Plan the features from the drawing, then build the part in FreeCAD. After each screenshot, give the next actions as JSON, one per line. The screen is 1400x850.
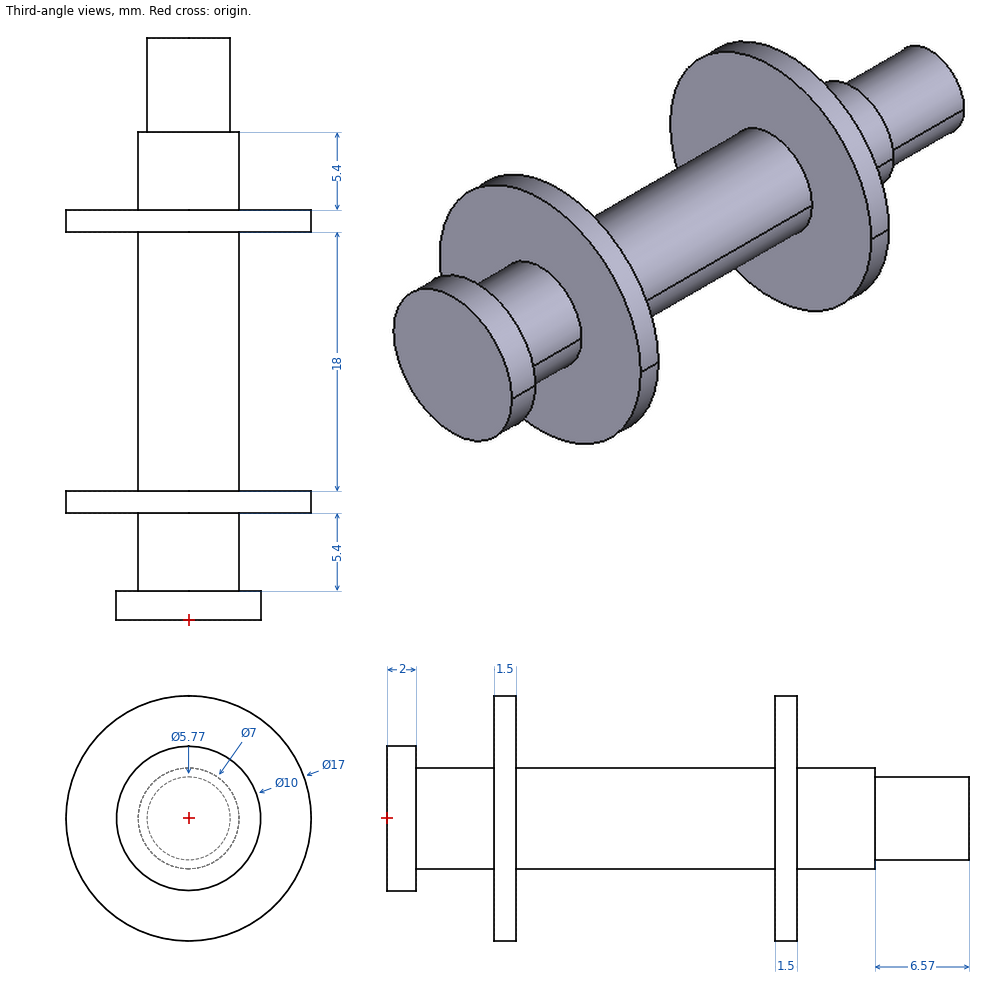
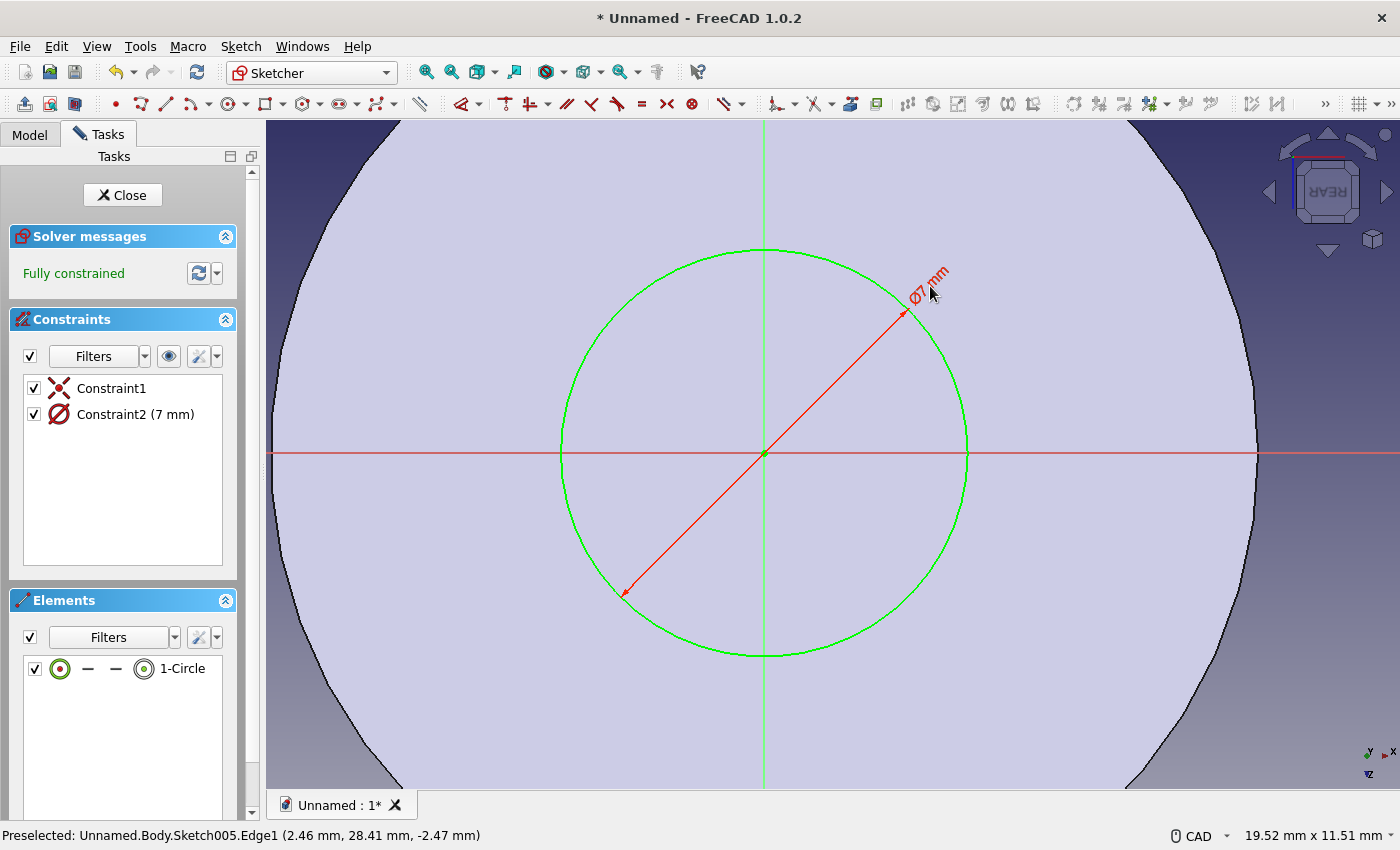
{"action": "left_click", "coordinate": [123, 195]}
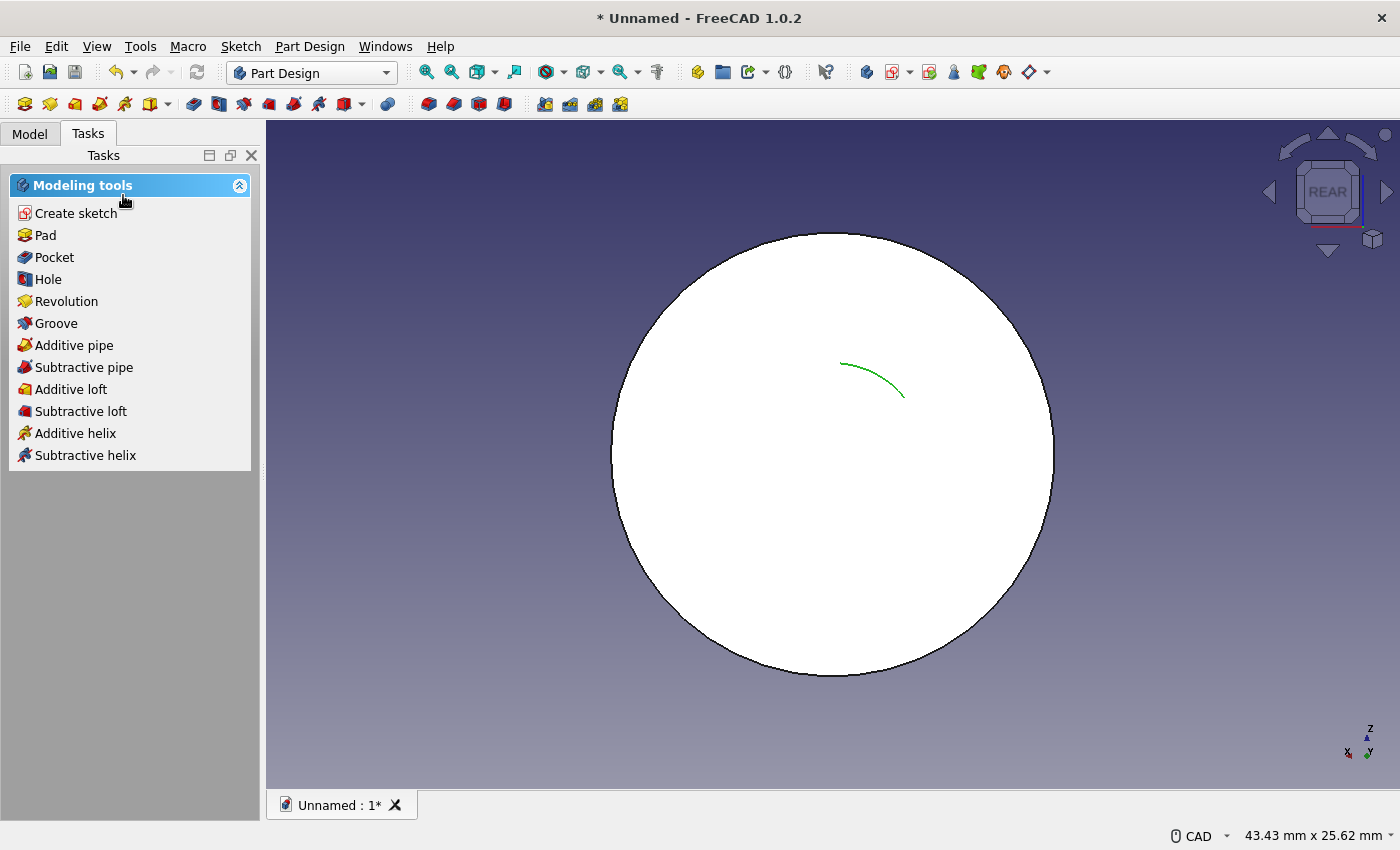
{"action": "left_click", "coordinate": [25, 104]}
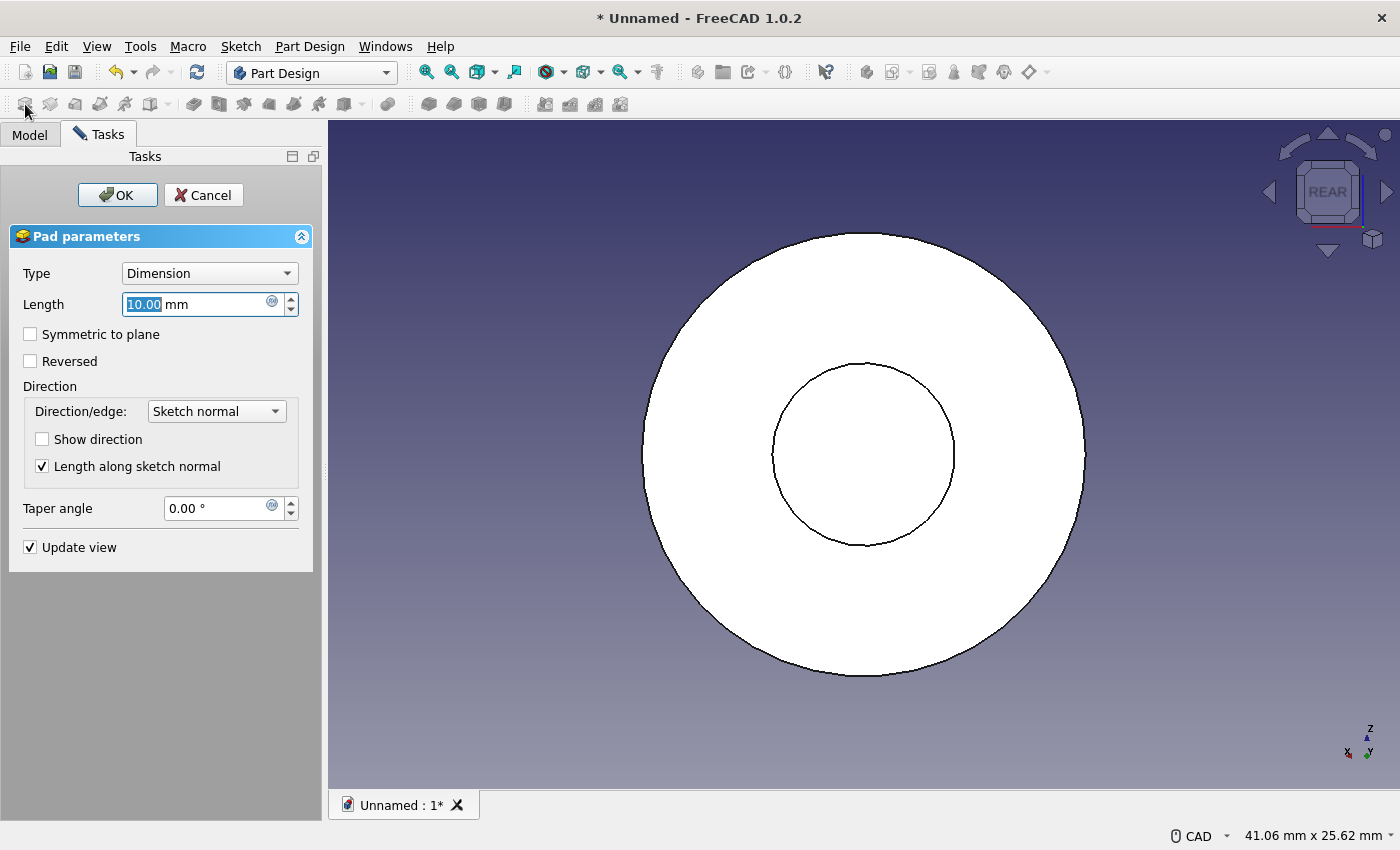
{"action": "type", "text": "5.4"}
{"action": "key", "text": "Tab"}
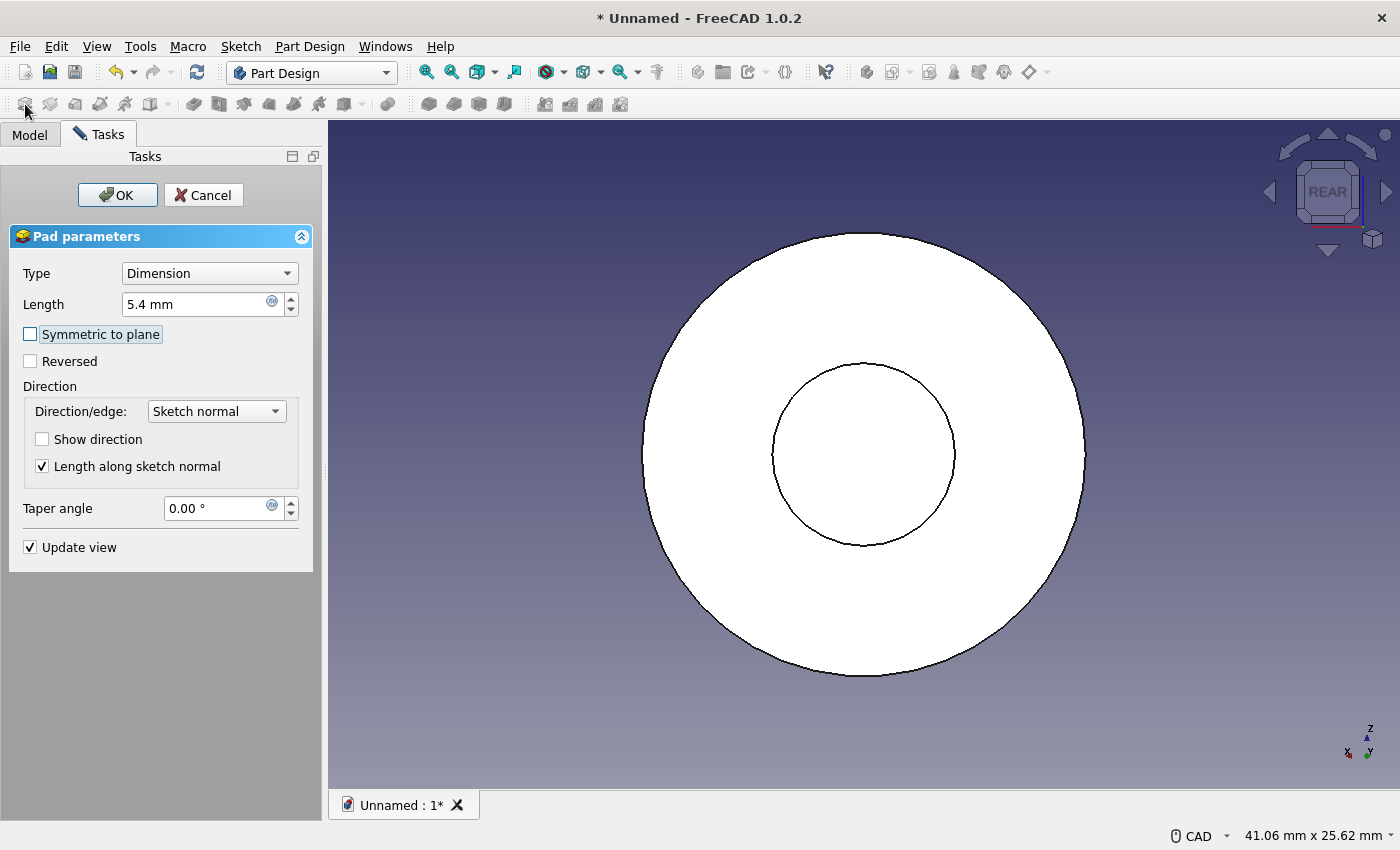
{"action": "left_click", "coordinate": [118, 195]}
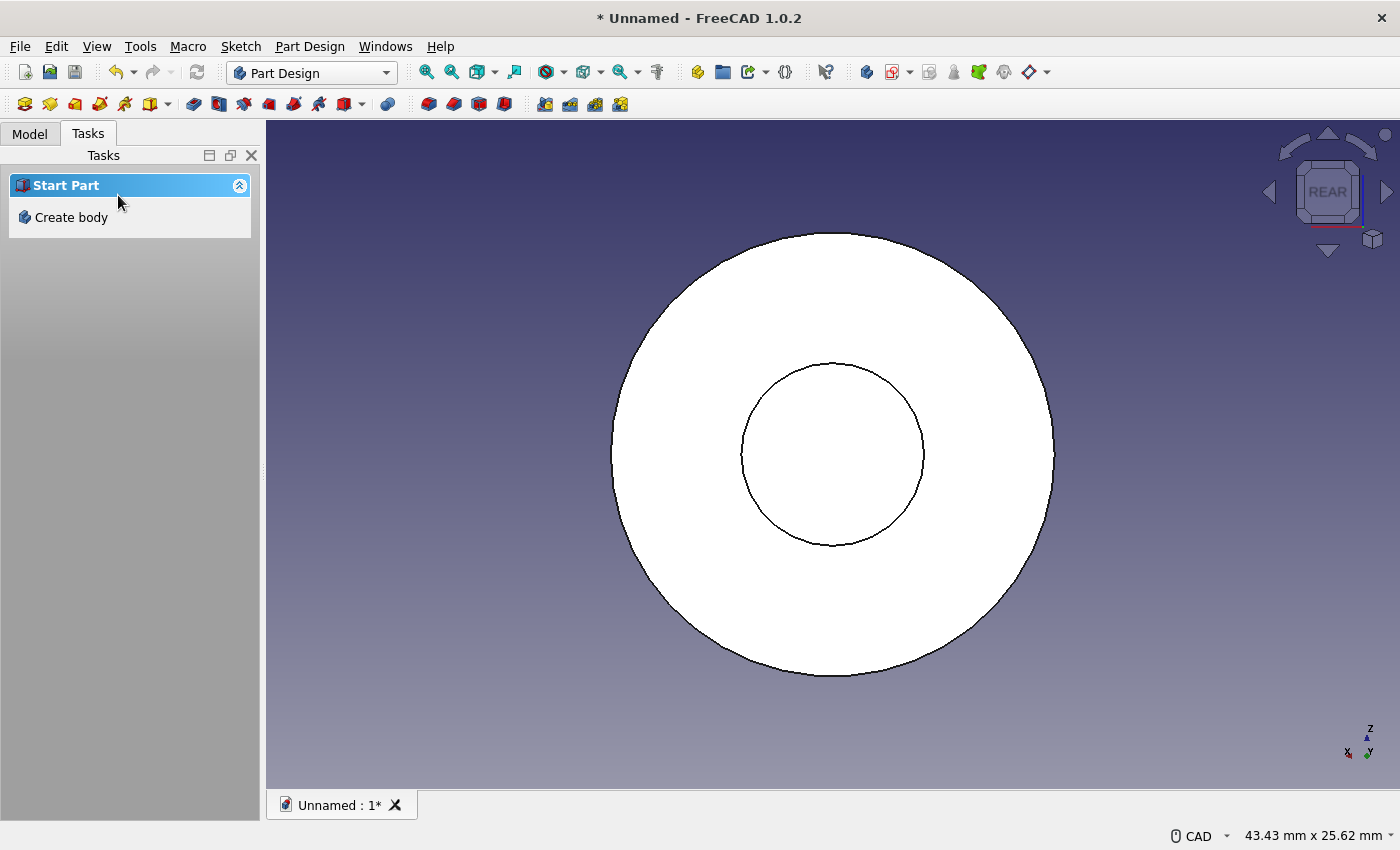
{"action": "left_click", "coordinate": [833, 453]}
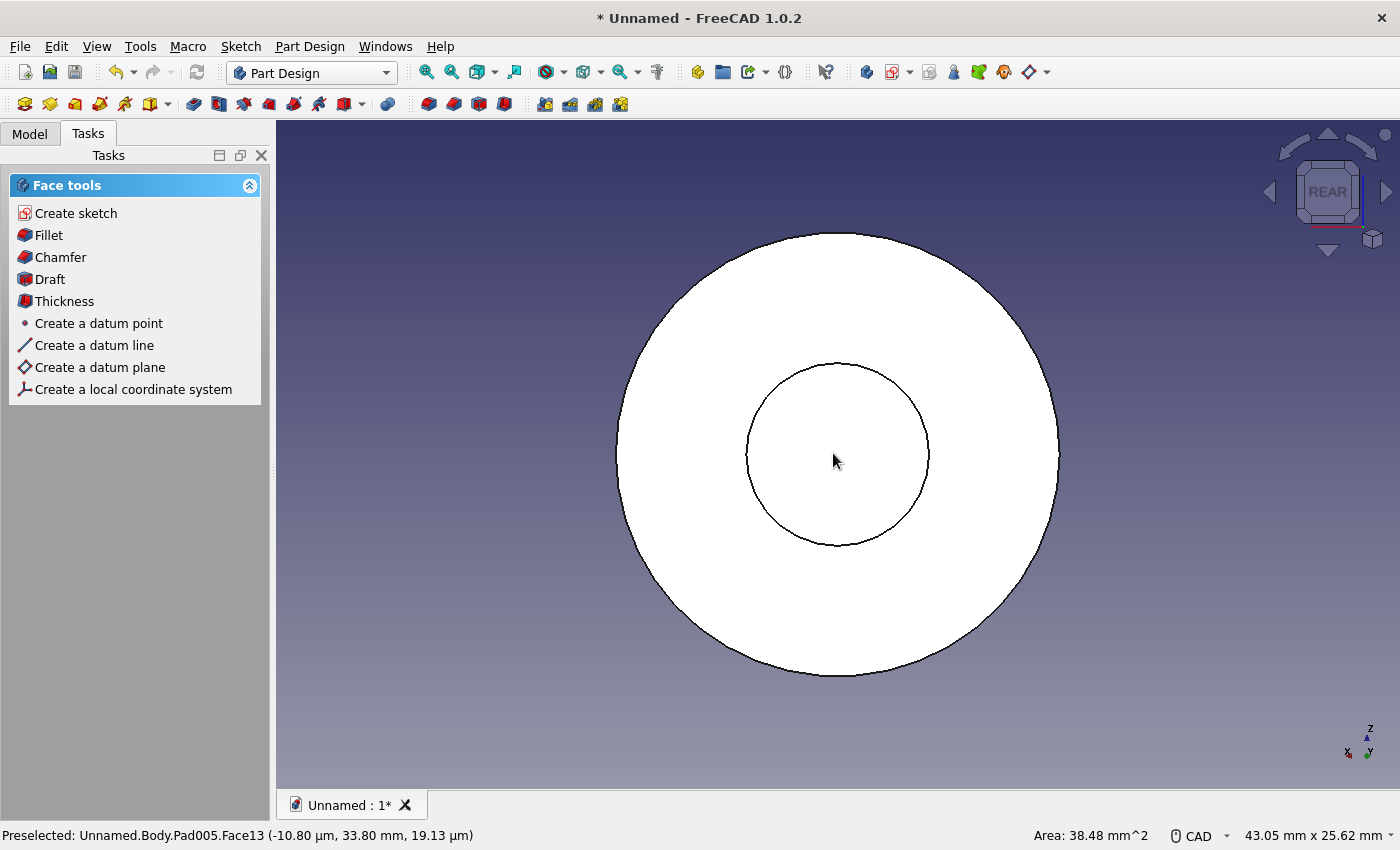
{"action": "left_click", "coordinate": [892, 72]}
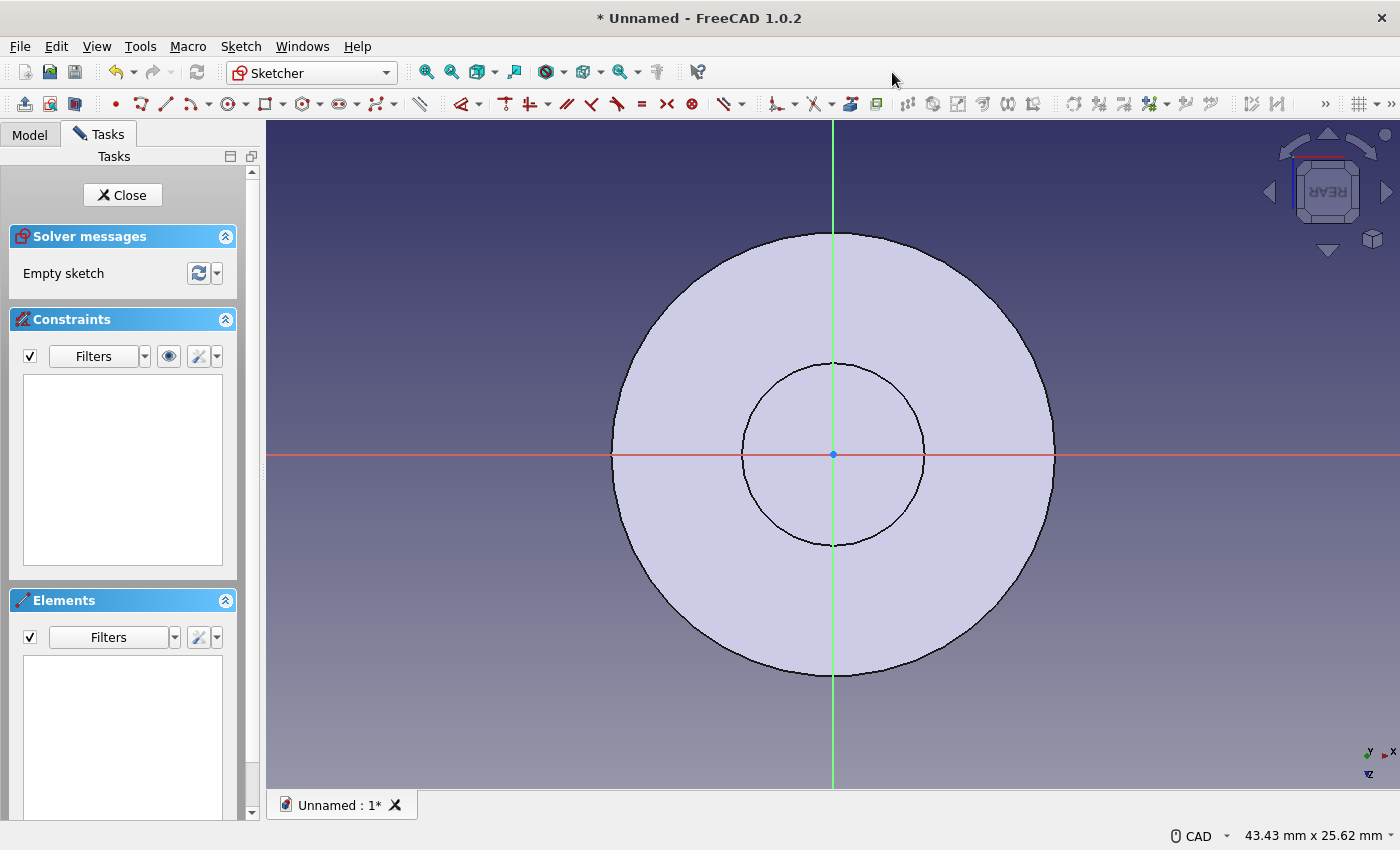
{"action": "scroll", "coordinate": [873, 455], "scroll_direction": "up", "scroll_amount": 5}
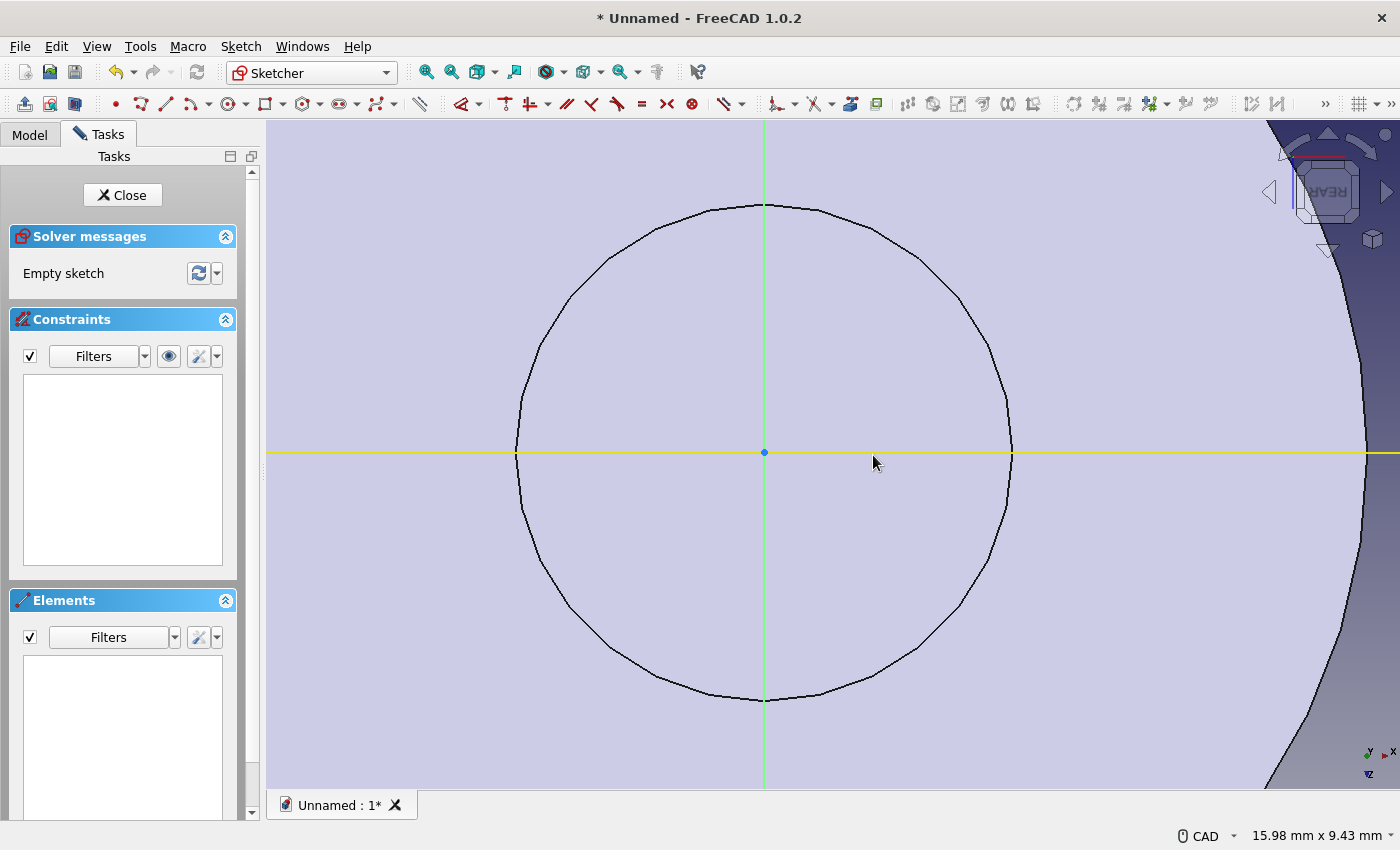
{"action": "left_click", "coordinate": [228, 104]}